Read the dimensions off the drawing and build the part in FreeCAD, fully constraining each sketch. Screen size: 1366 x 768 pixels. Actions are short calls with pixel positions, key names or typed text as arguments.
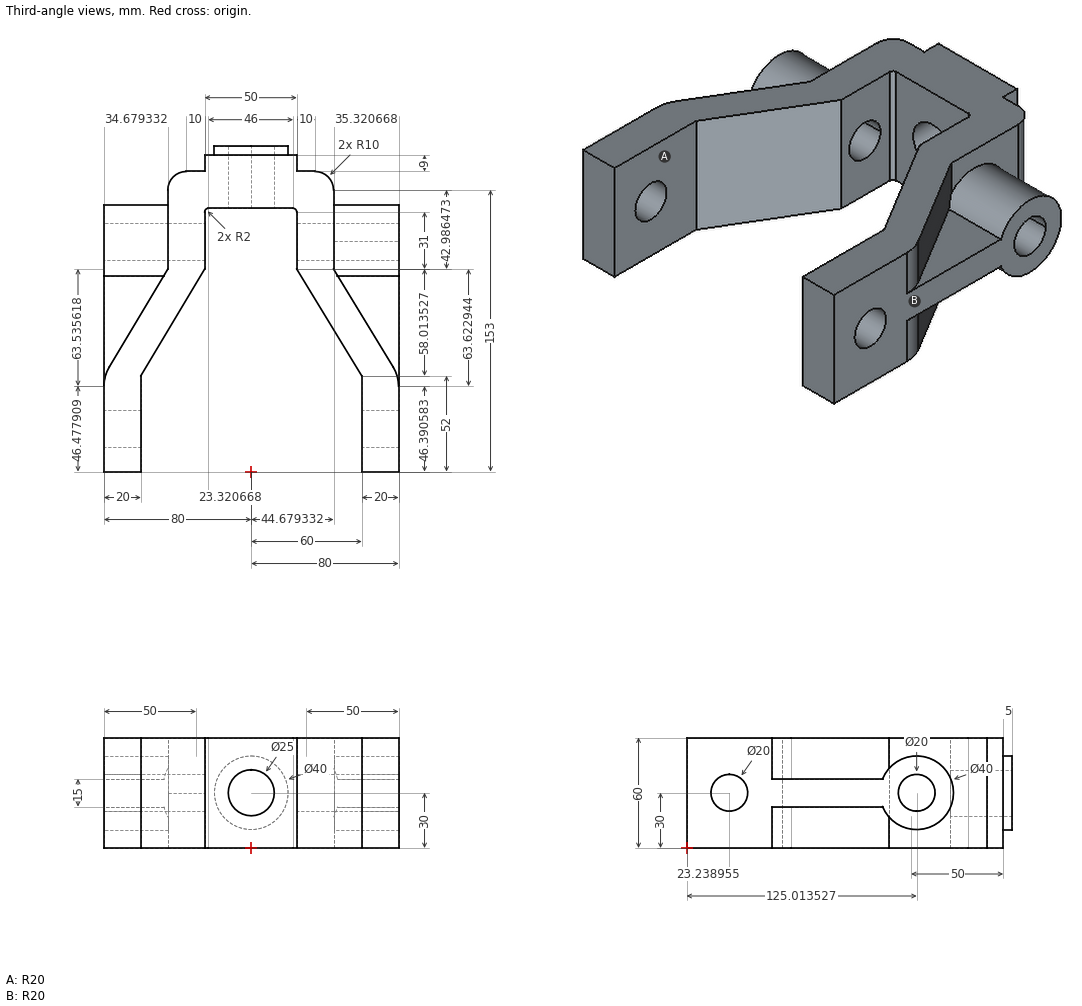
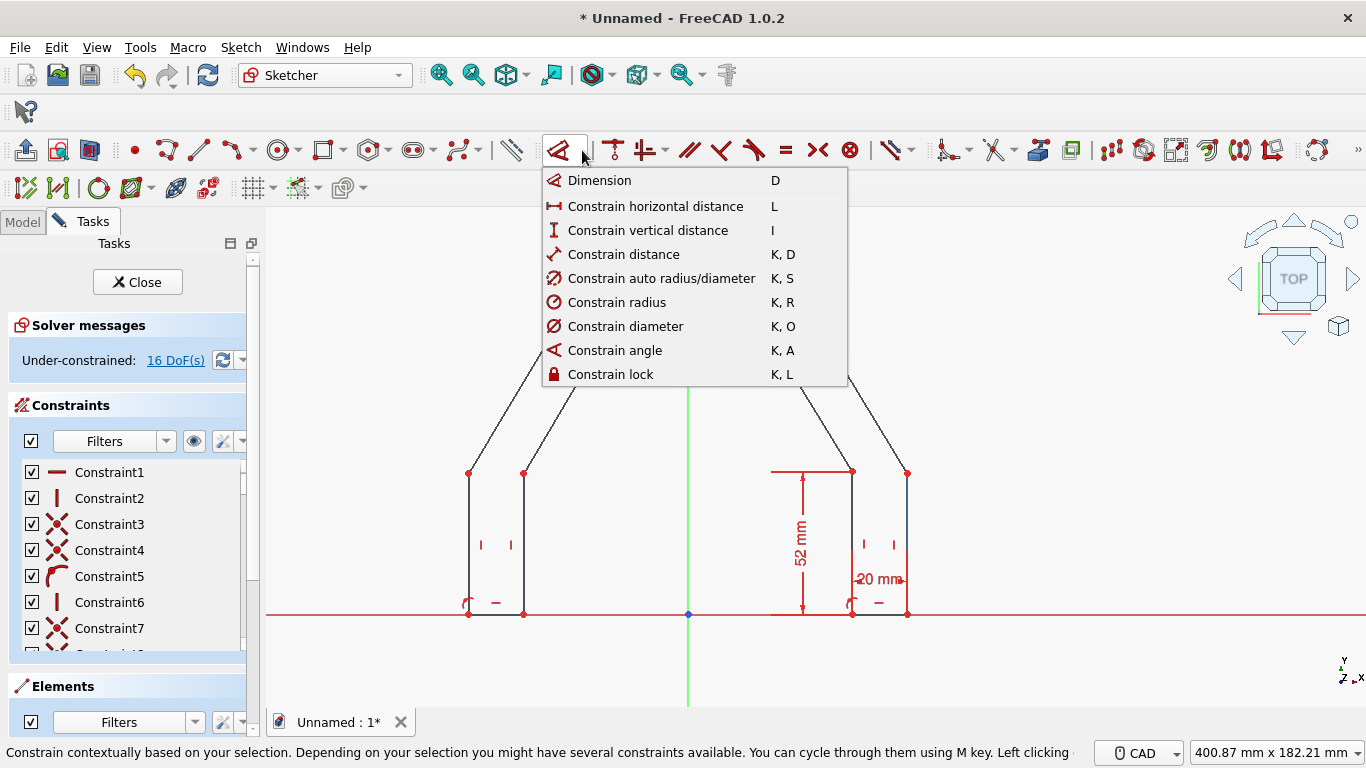
click(695, 230)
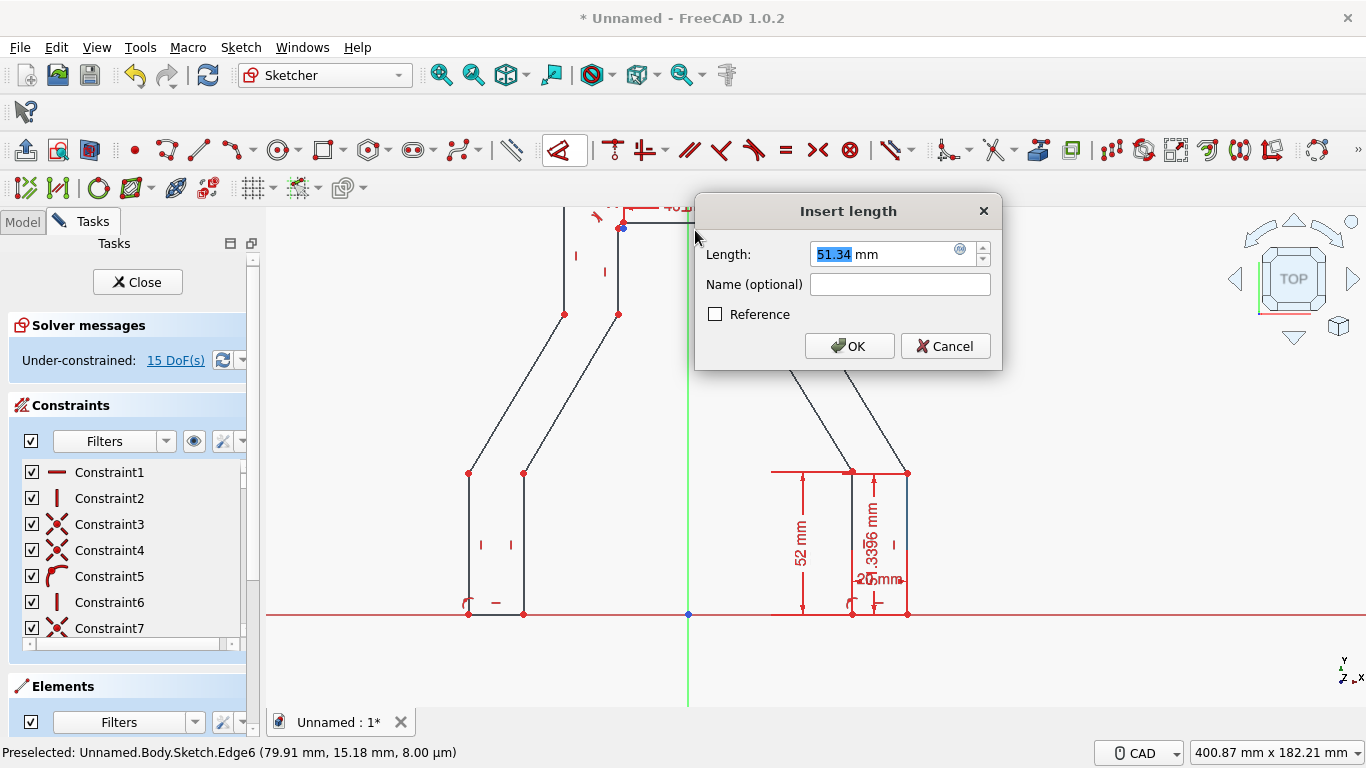
text(52)
key(Return)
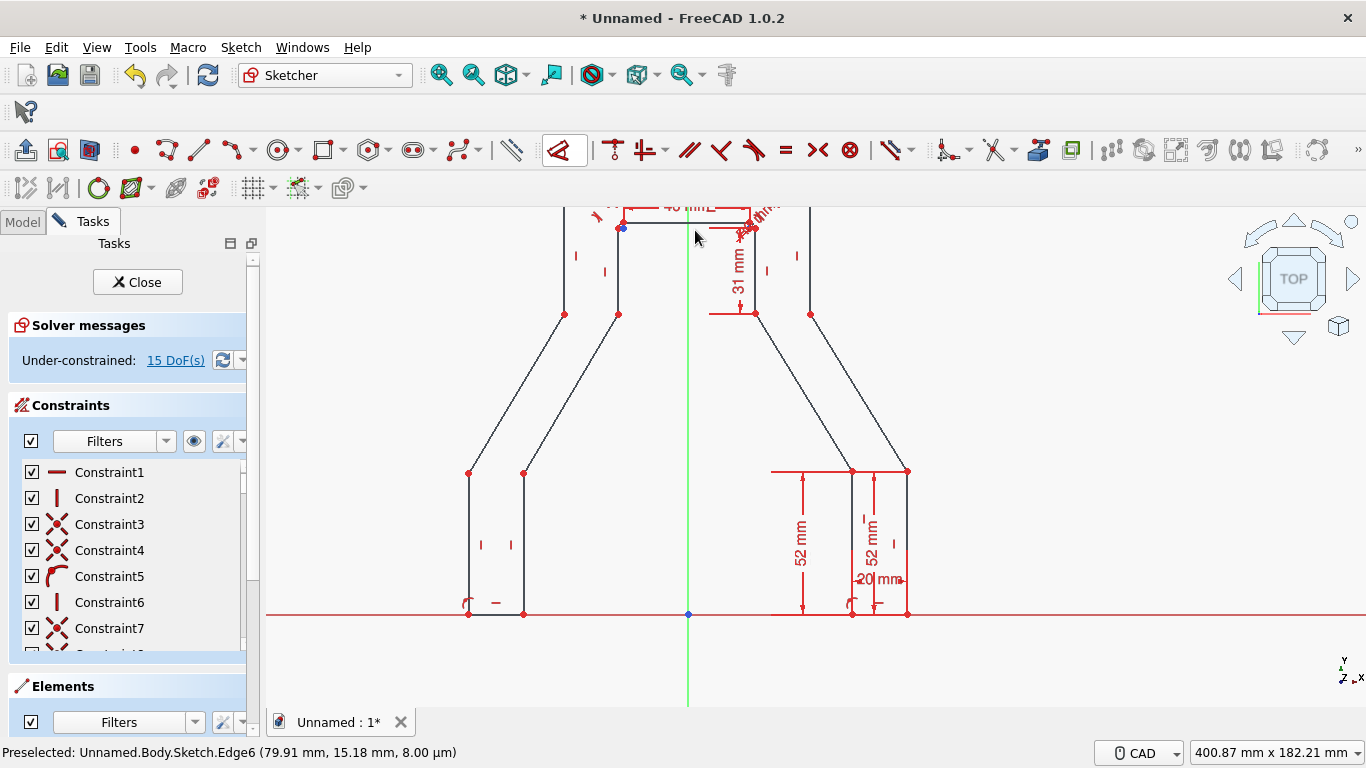
scroll(868, 616, down, 2)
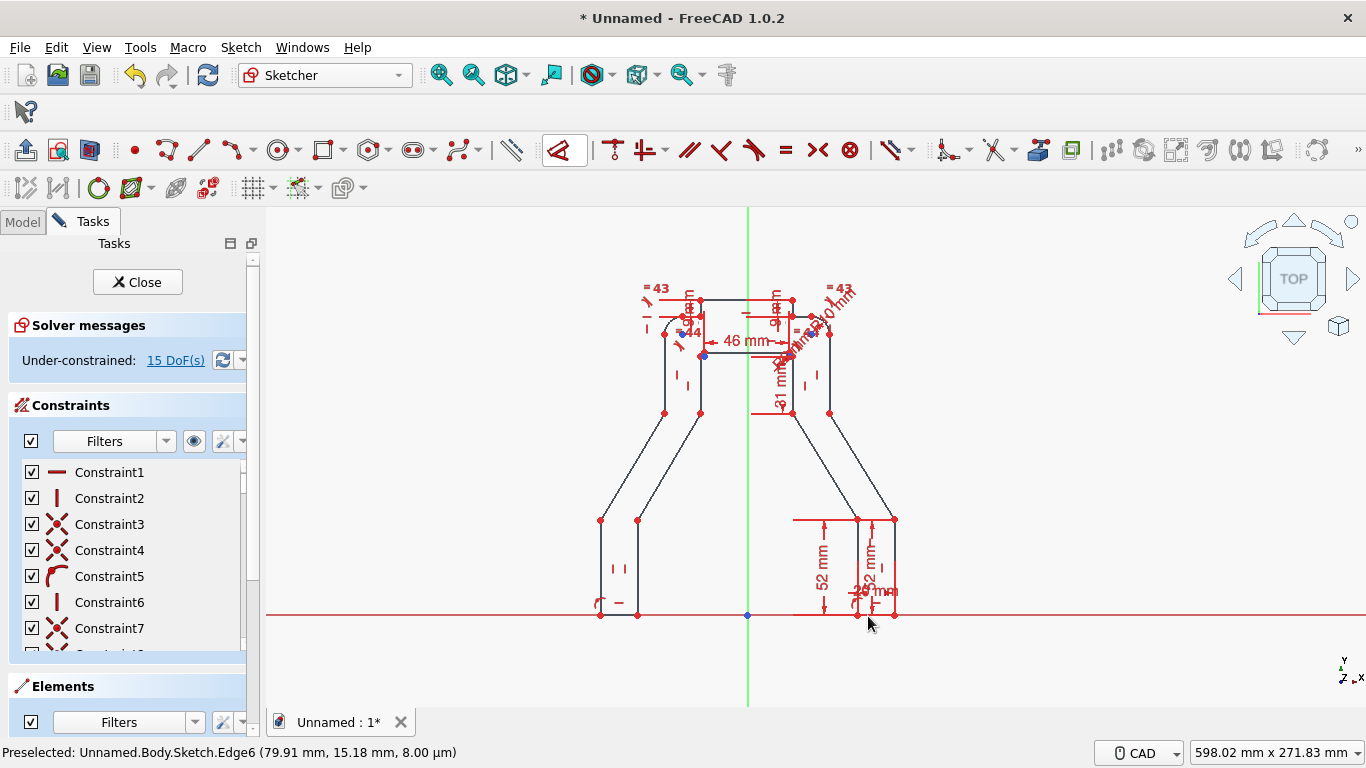
scroll(804, 317, up, 4)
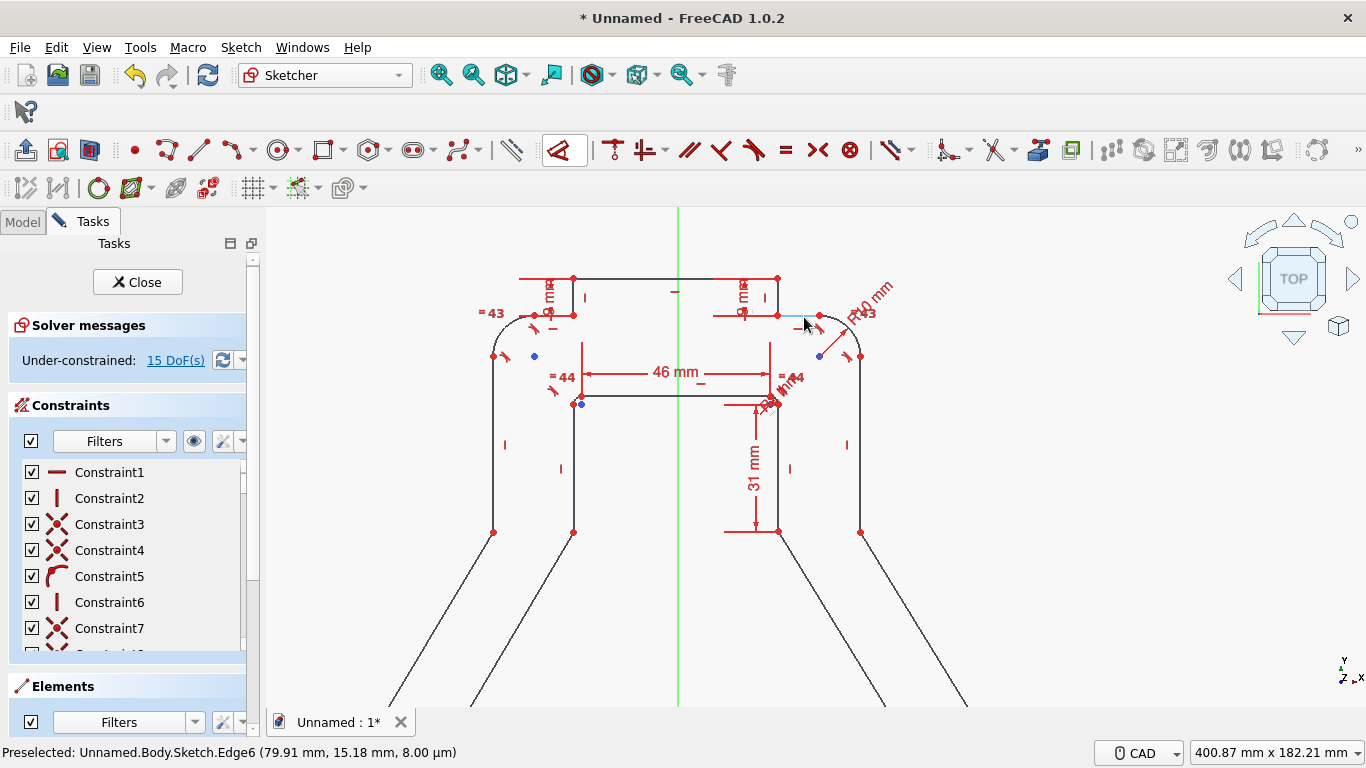
click(803, 316)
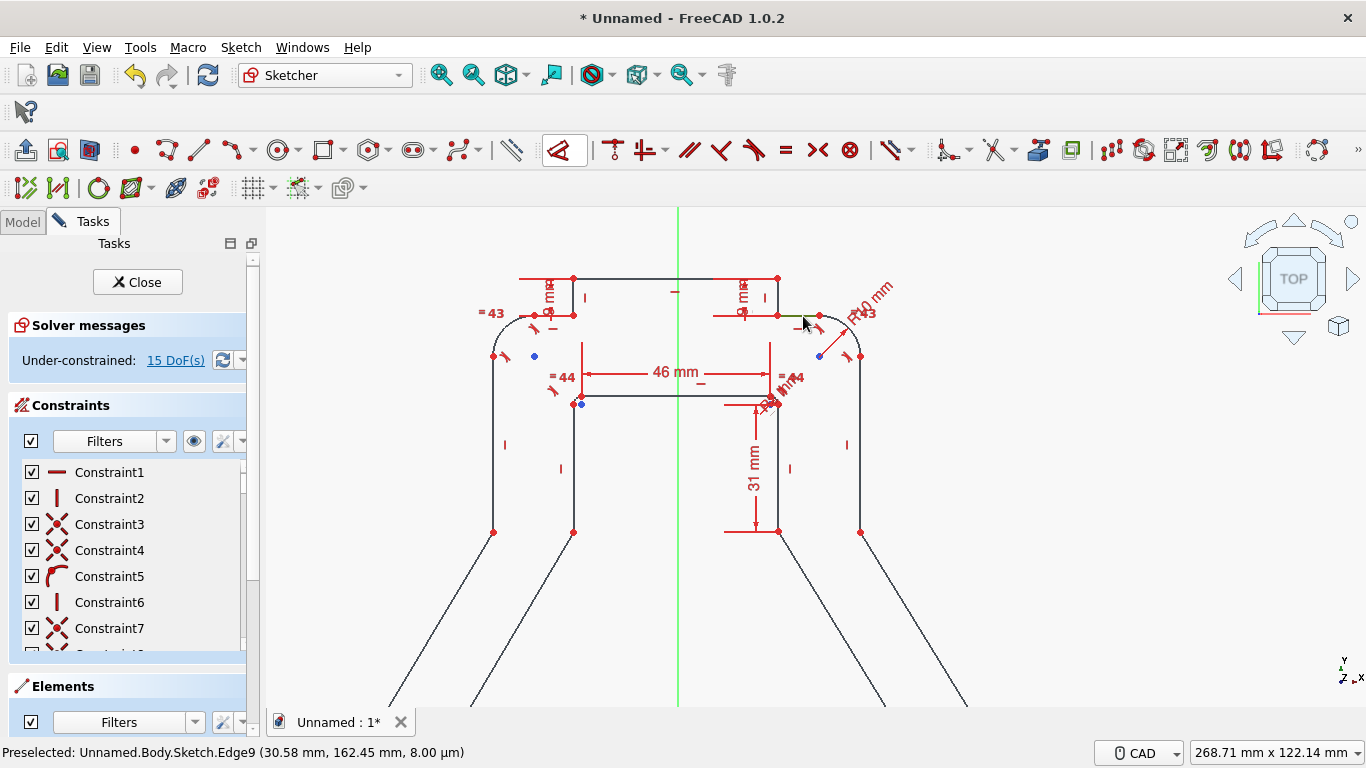
key(l)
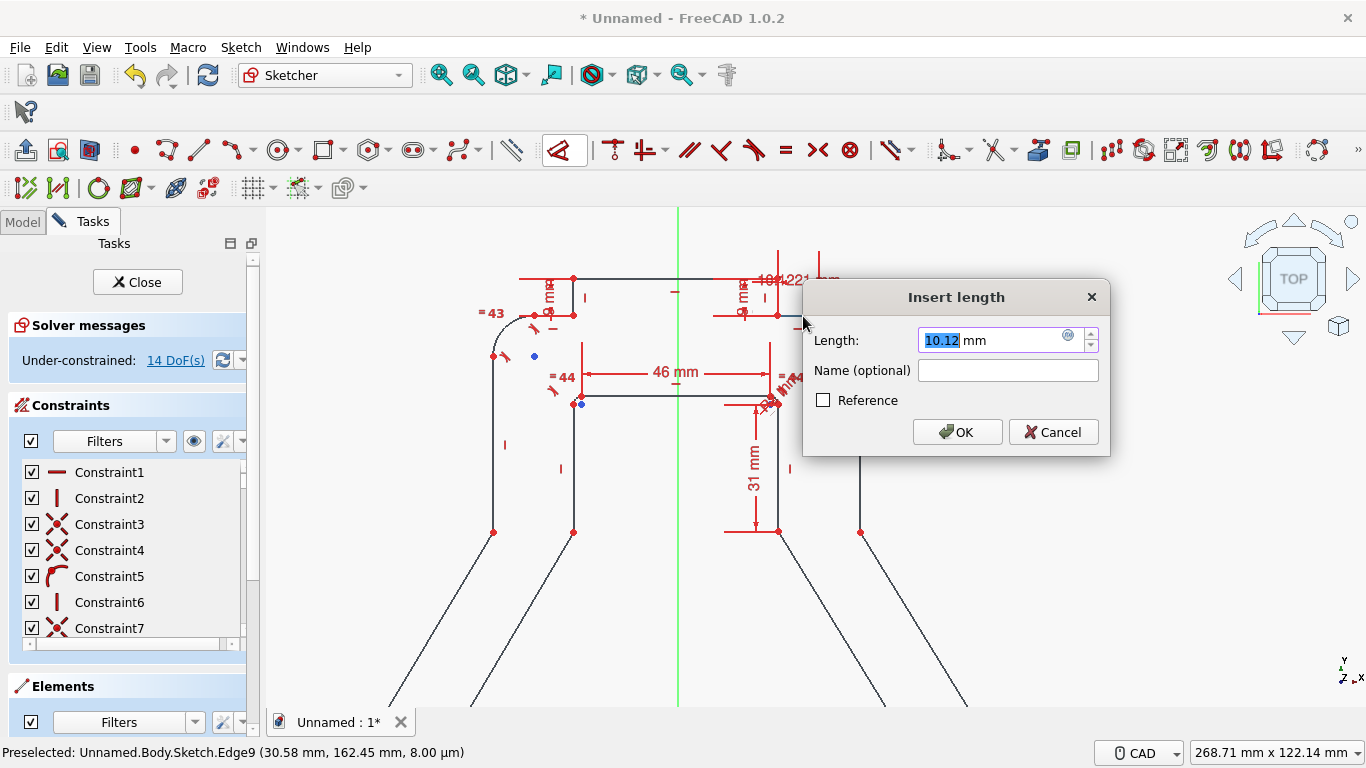
text(10)
key(Return)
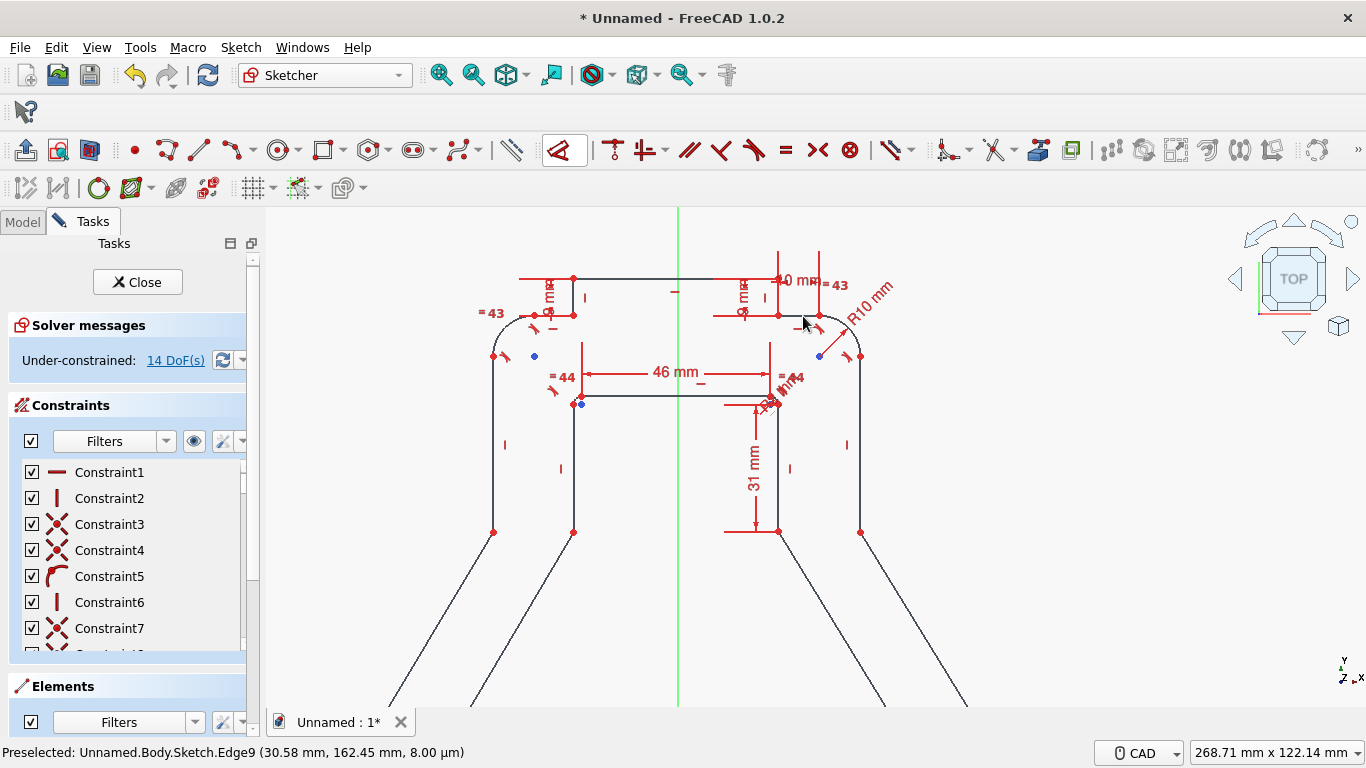
click(717, 279)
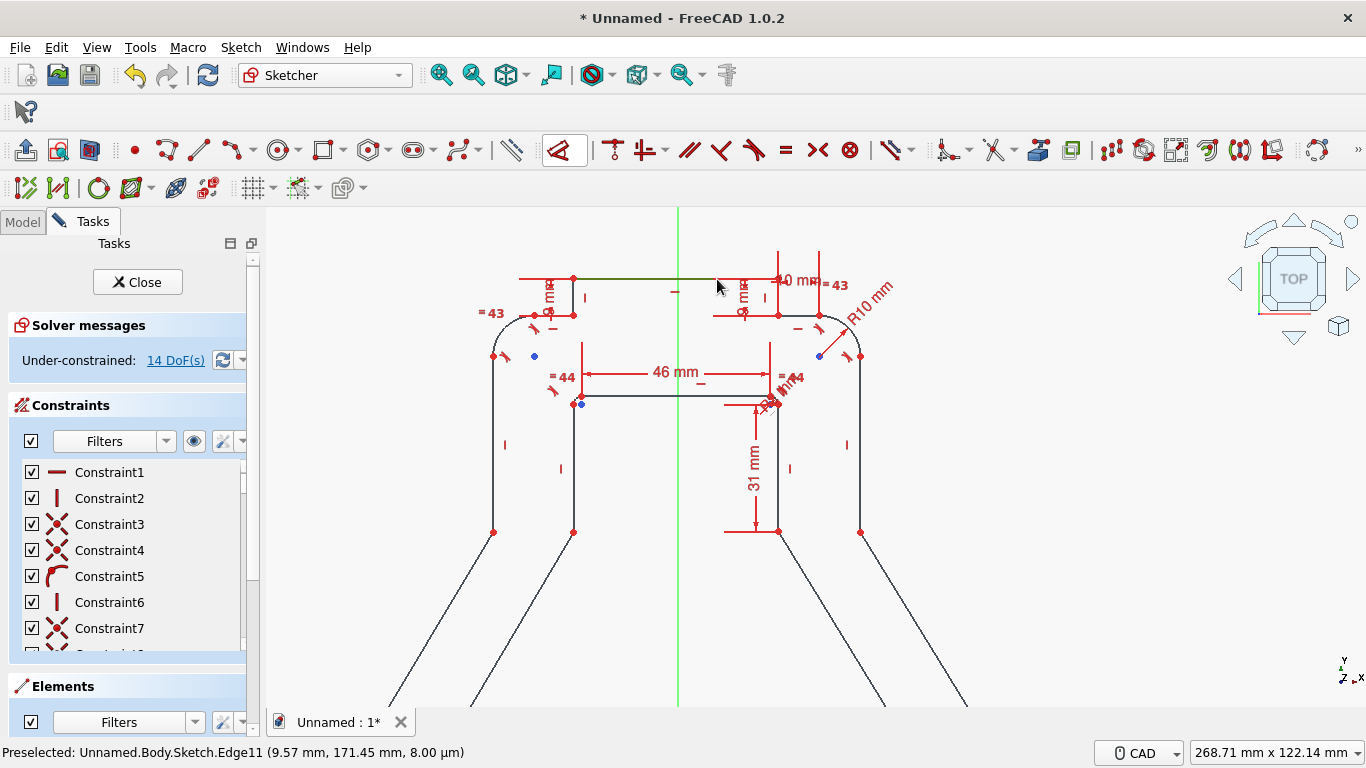
key(l)